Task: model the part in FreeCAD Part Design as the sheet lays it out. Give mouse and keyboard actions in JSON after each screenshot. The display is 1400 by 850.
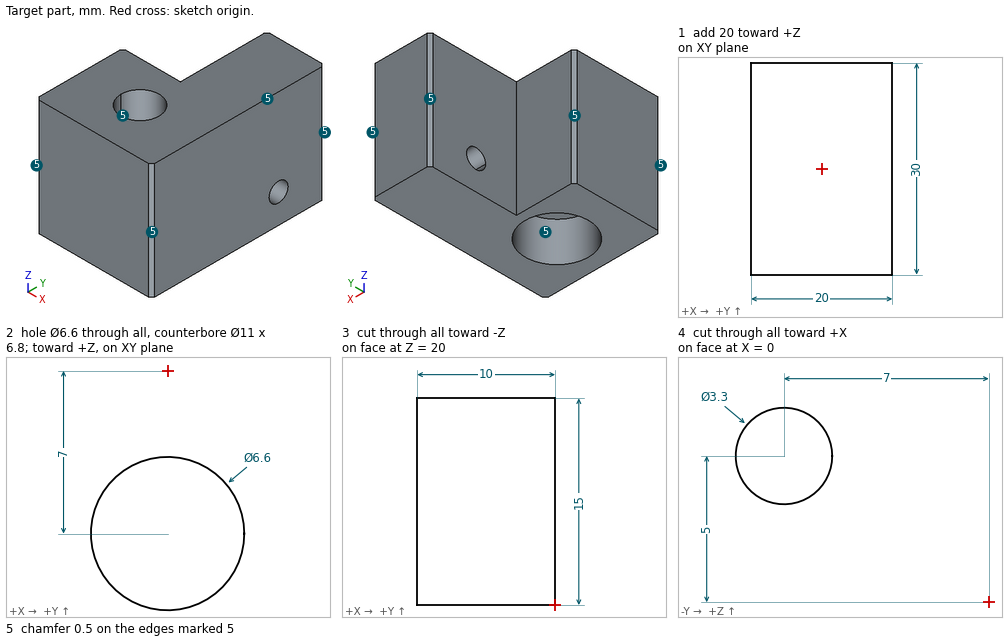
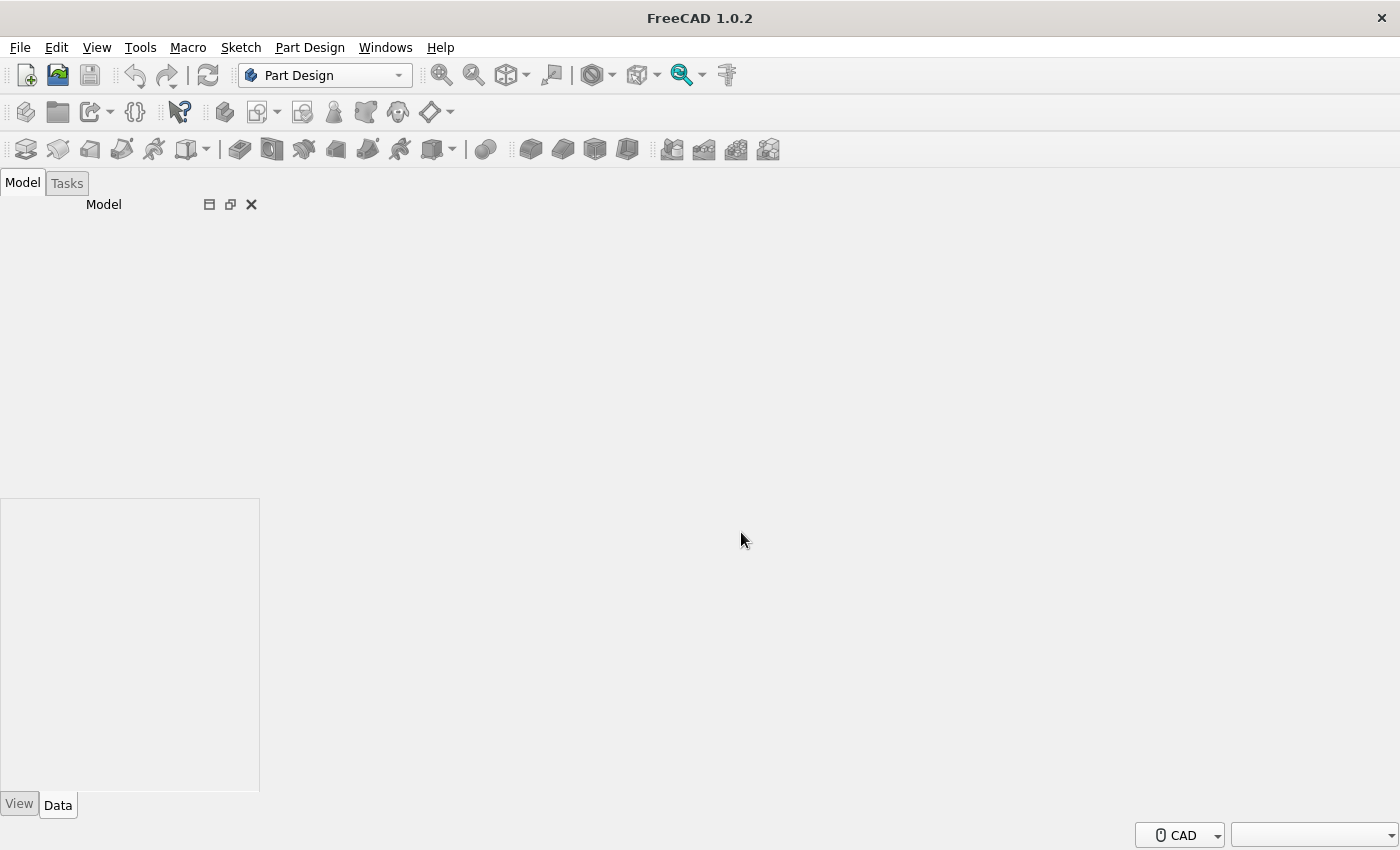
{"action": "left_click", "coordinate": [26, 76]}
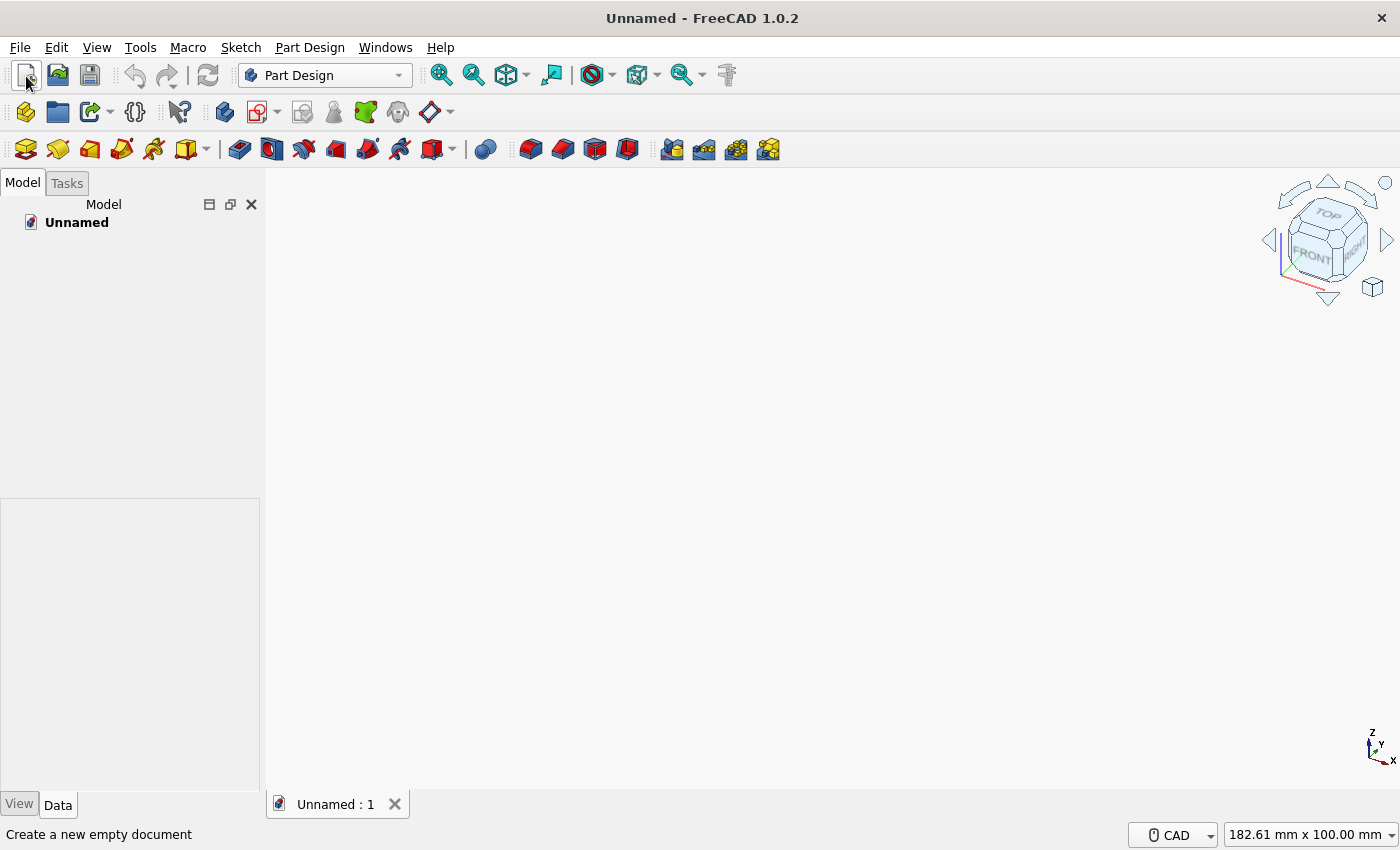
{"action": "left_click", "coordinate": [258, 112]}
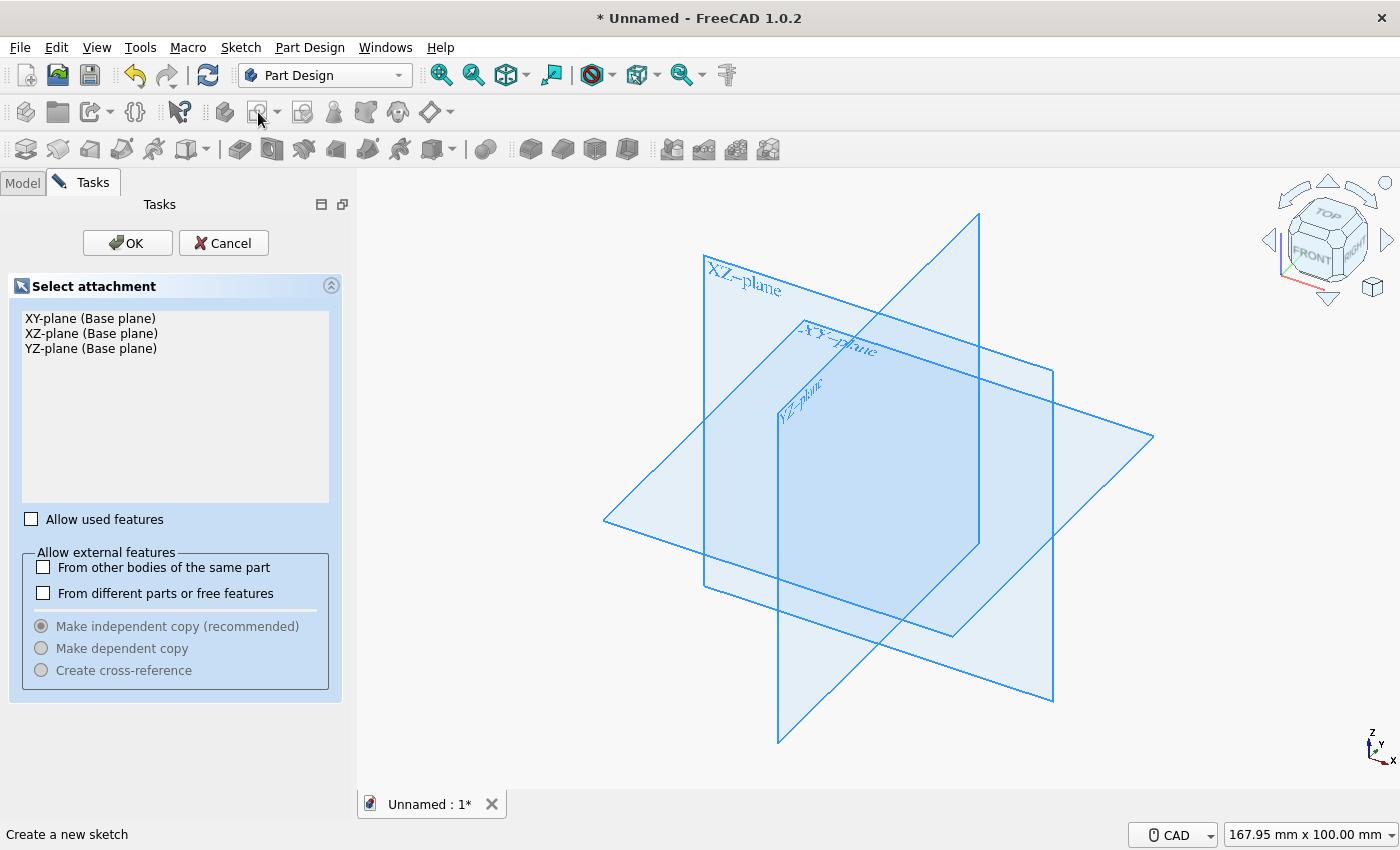
{"action": "left_click", "coordinate": [82, 318]}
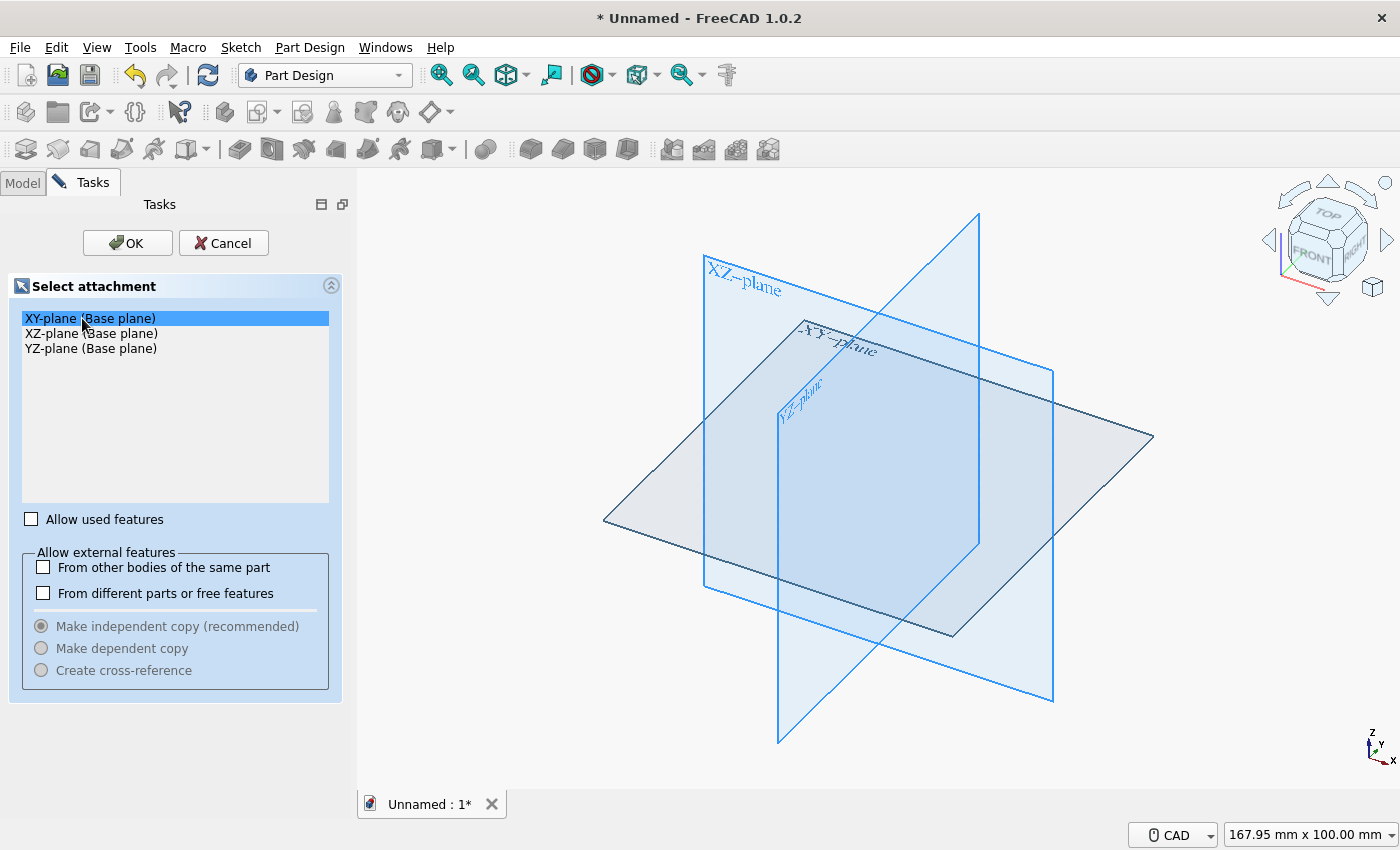
{"action": "left_click", "coordinate": [128, 243]}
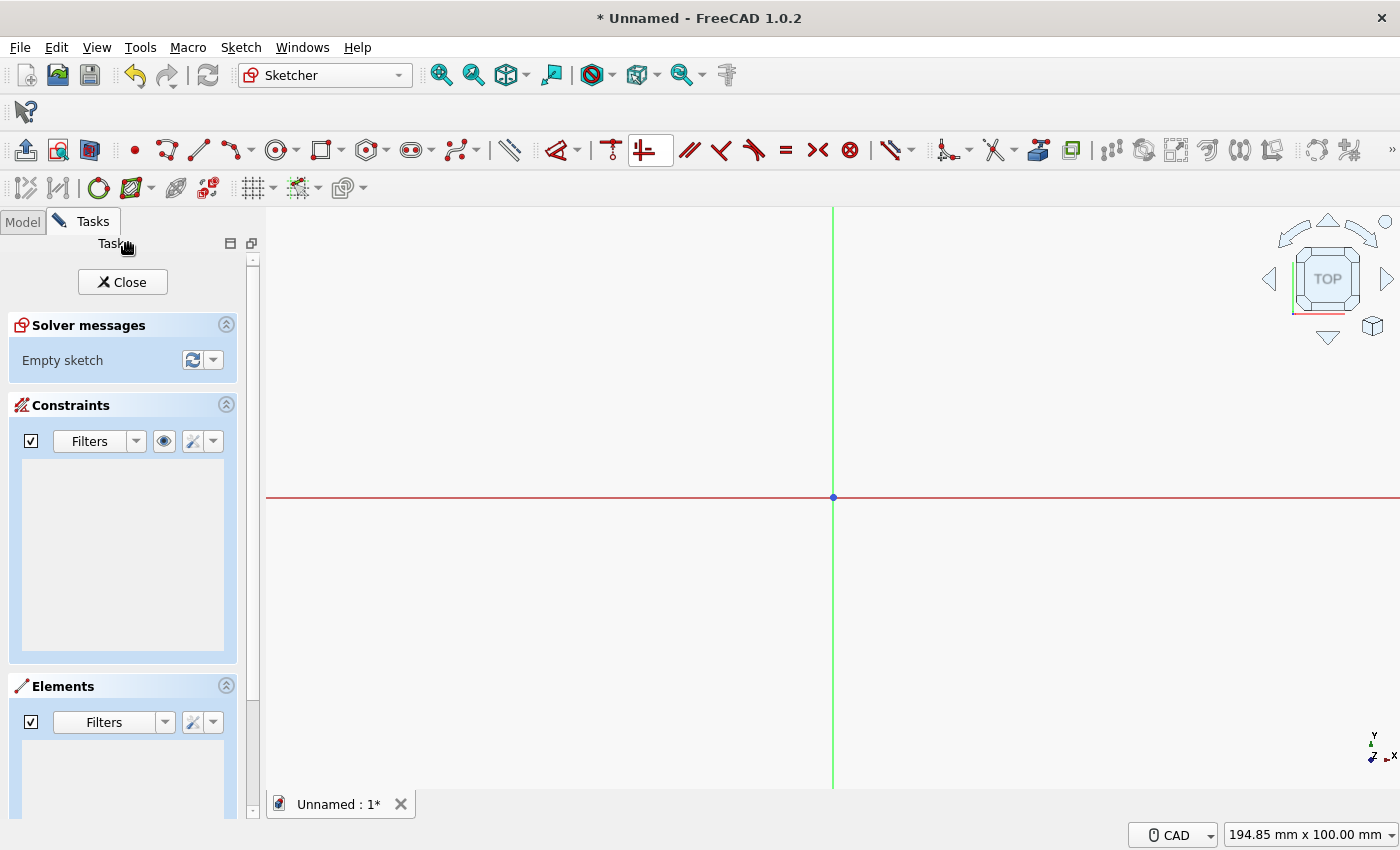
{"action": "scroll", "coordinate": [889, 498], "scroll_direction": "up", "scroll_amount": 4}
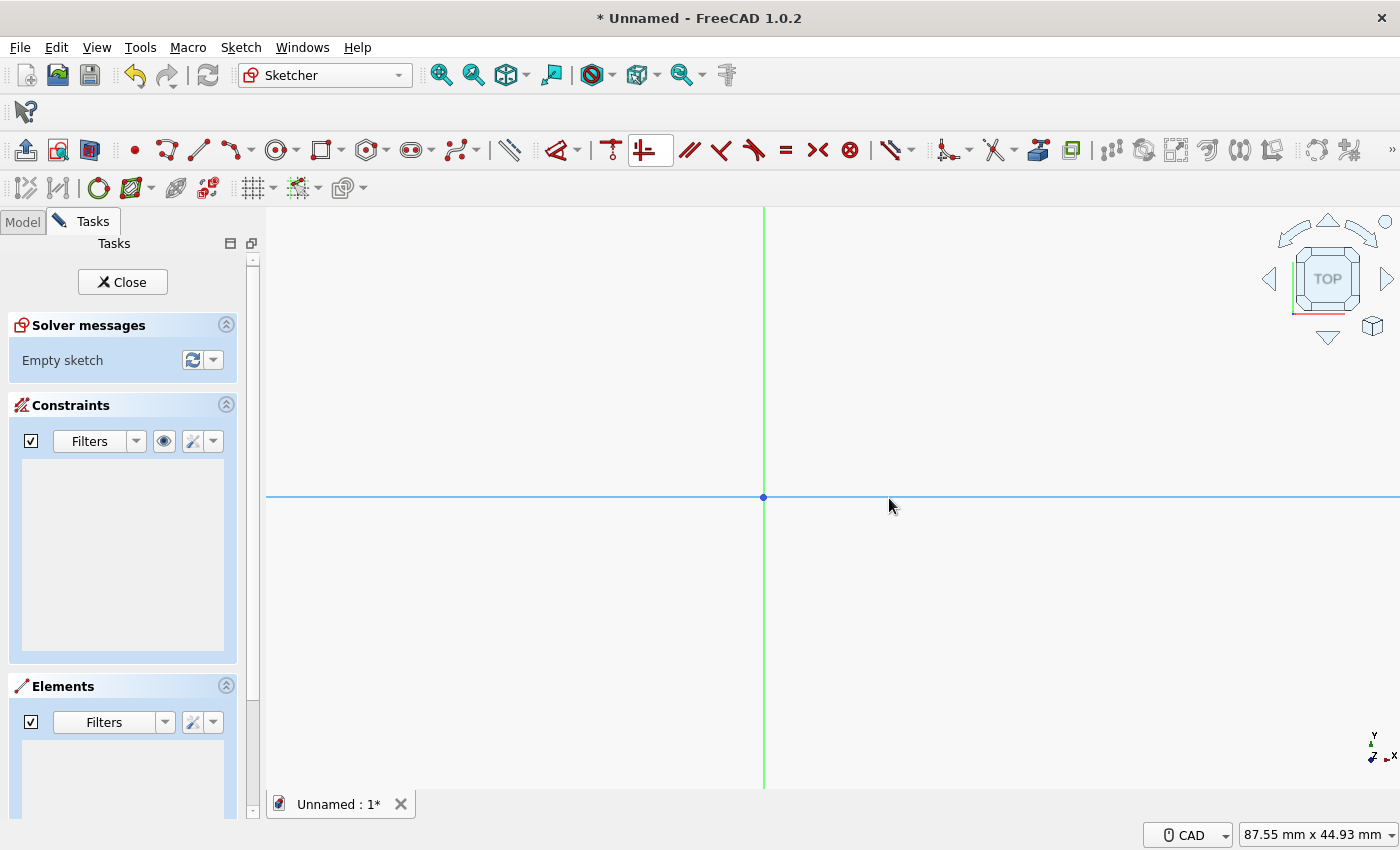
{"action": "left_click", "coordinate": [344, 150]}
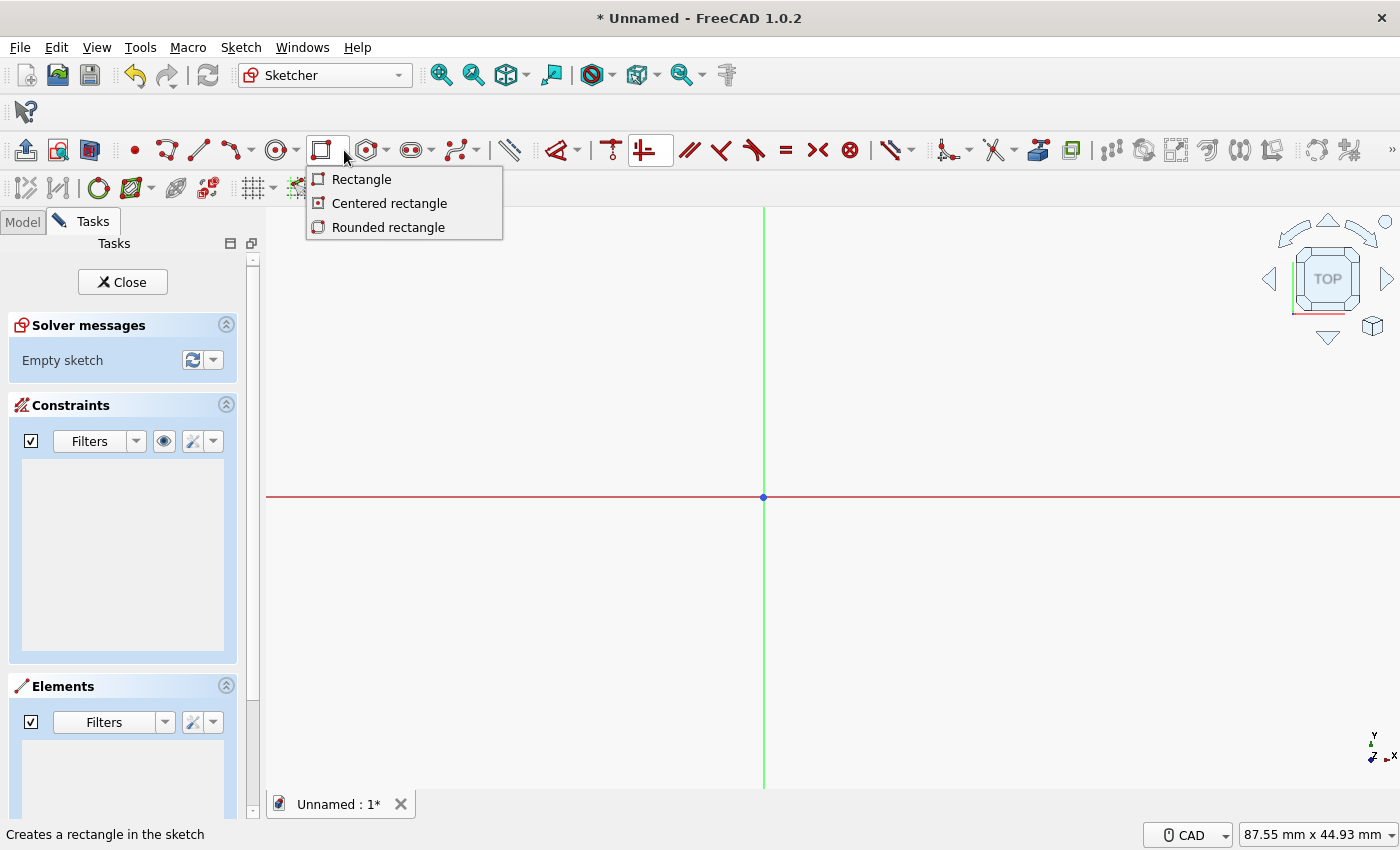
{"action": "left_click", "coordinate": [404, 203]}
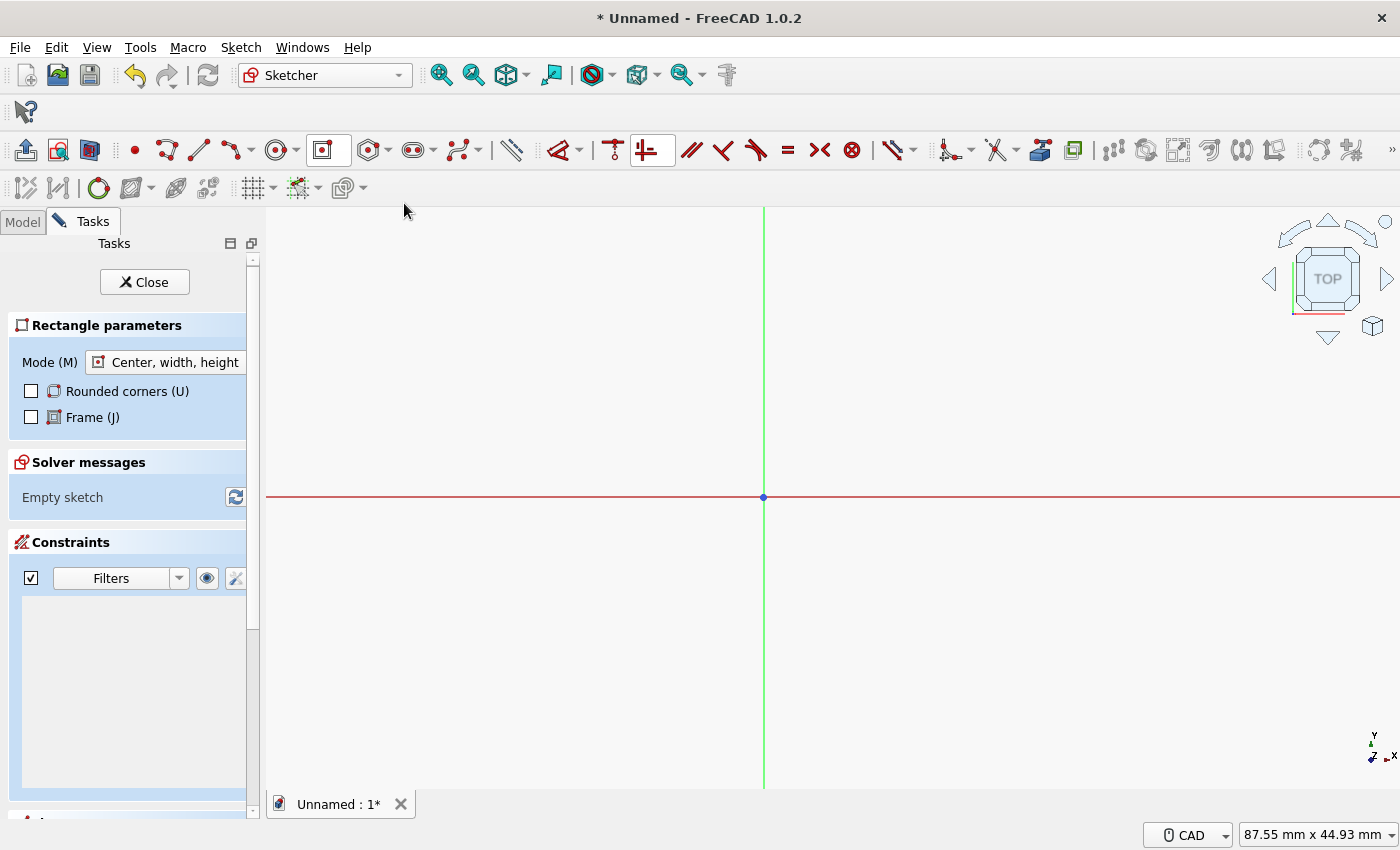
{"action": "left_click", "coordinate": [764, 497]}
{"action": "left_click", "coordinate": [893, 303]}
{"action": "key", "text": "Escape"}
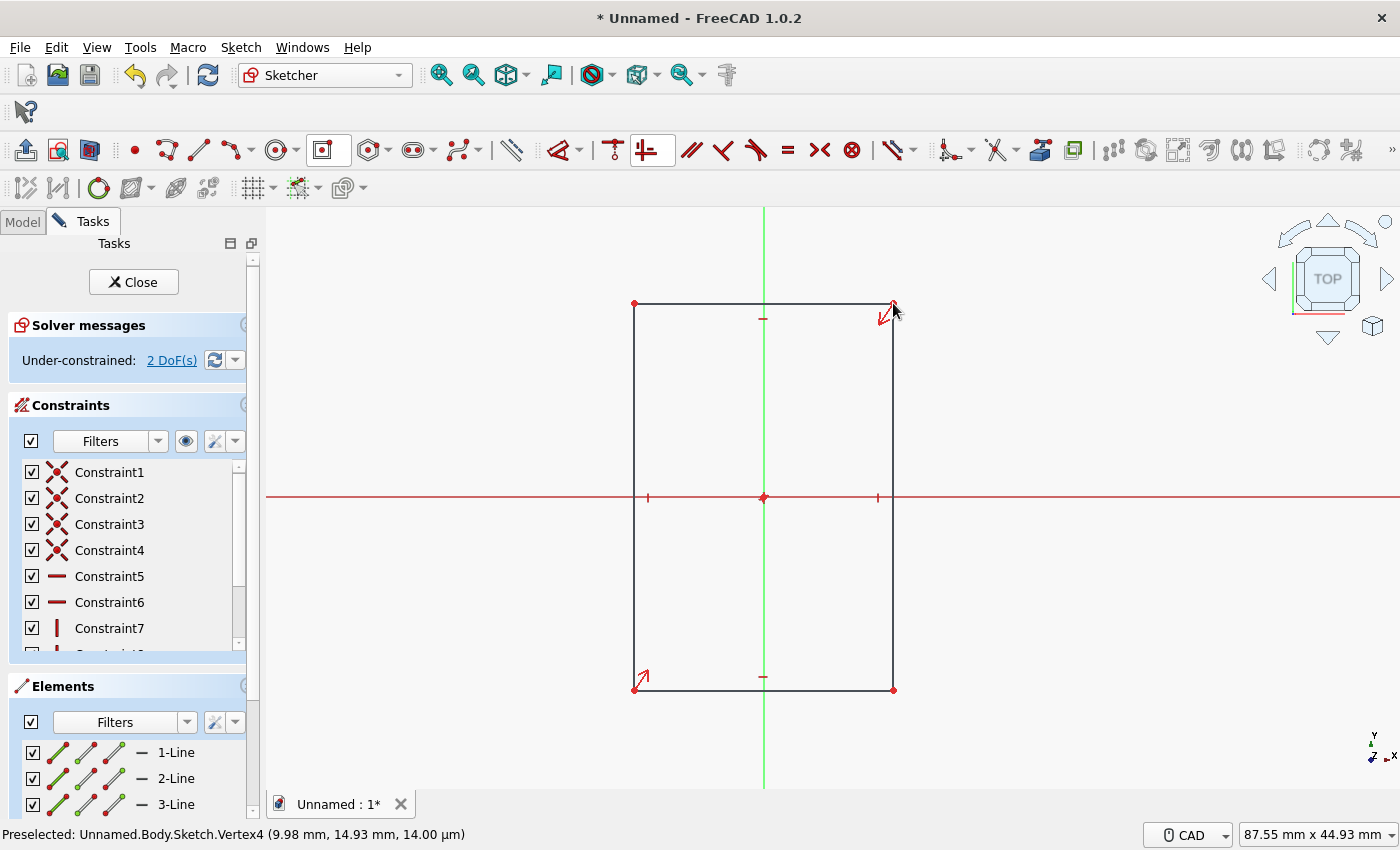
{"action": "left_click", "coordinate": [558, 150]}